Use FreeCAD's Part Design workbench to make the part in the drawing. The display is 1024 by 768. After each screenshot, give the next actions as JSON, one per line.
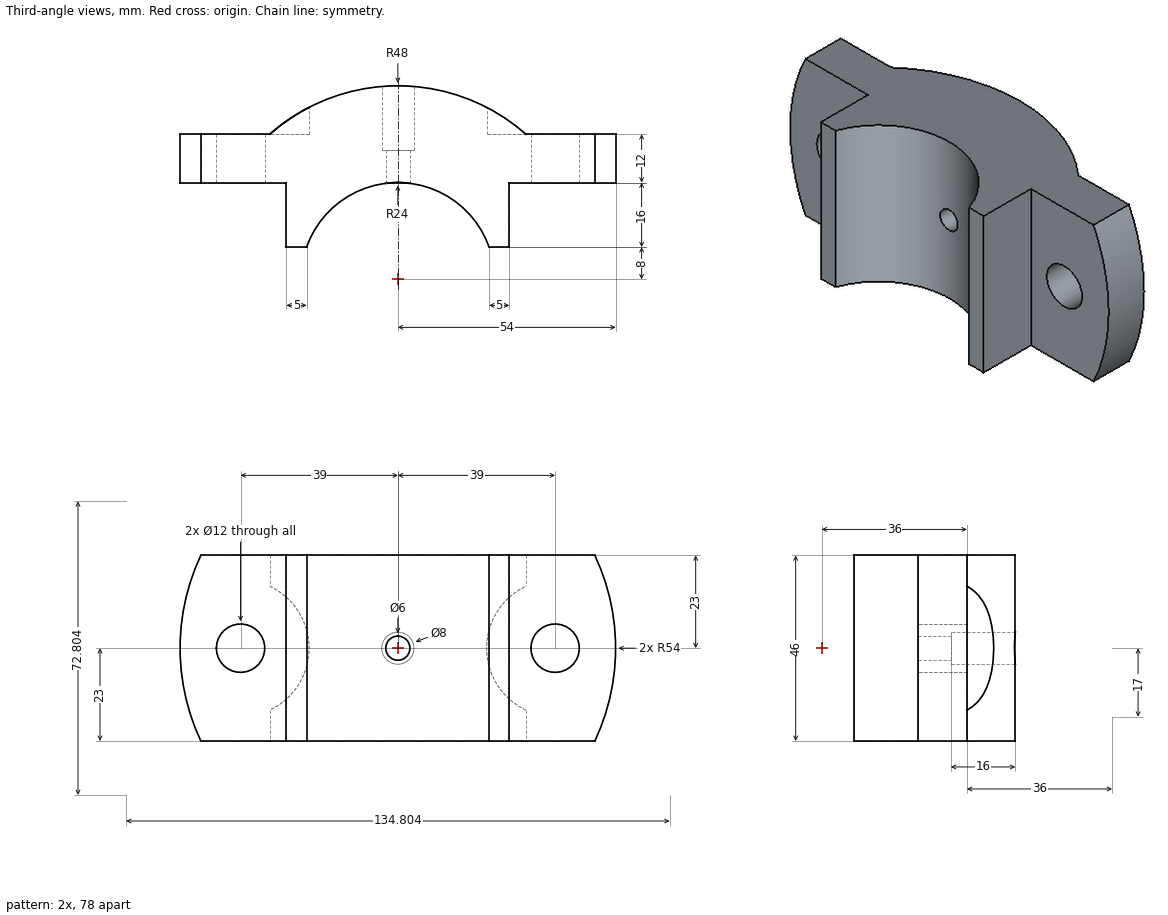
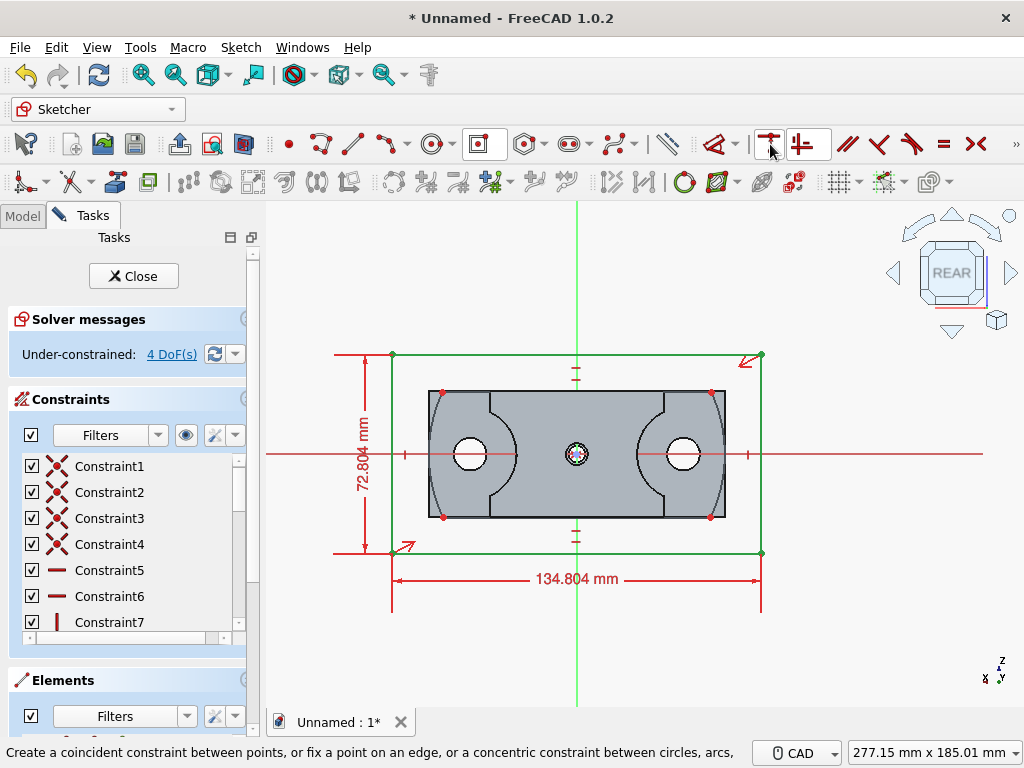
{"action": "left_click", "coordinate": [431, 429]}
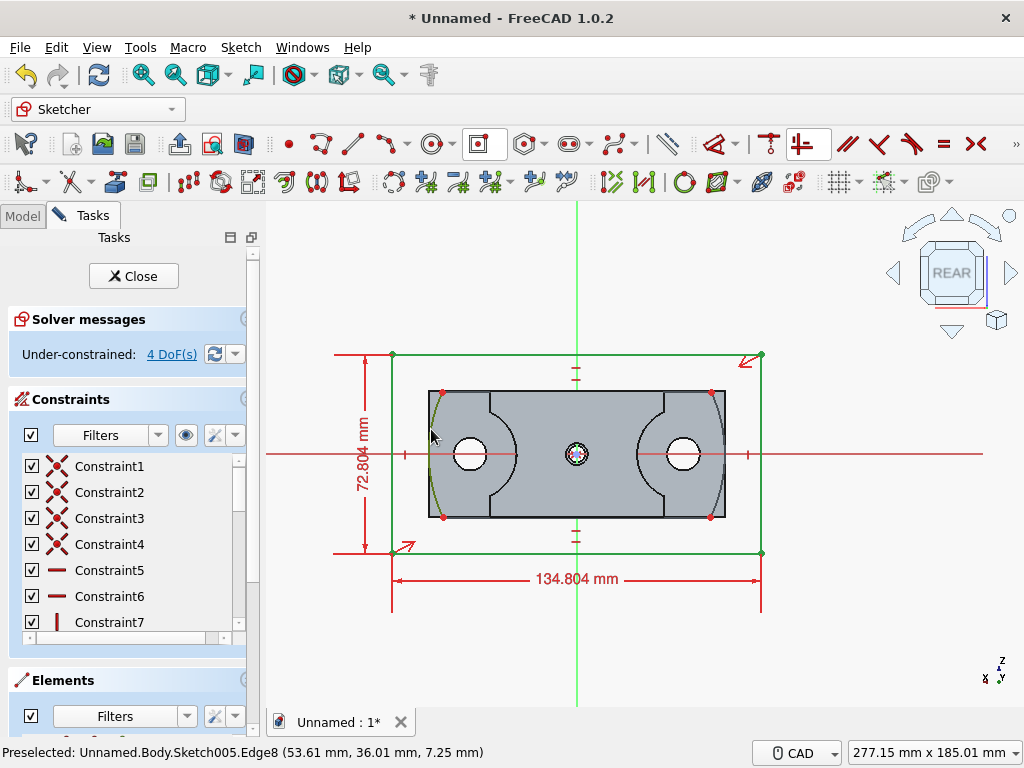
{"action": "left_click", "coordinate": [722, 481]}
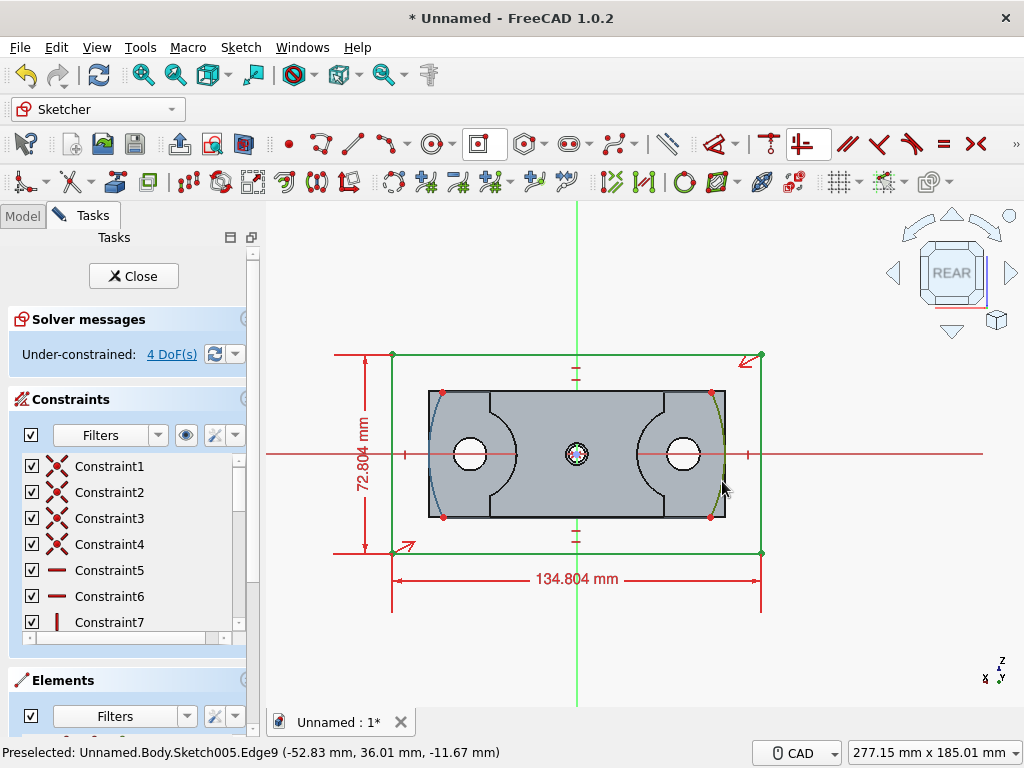
{"action": "left_click", "coordinate": [944, 144]}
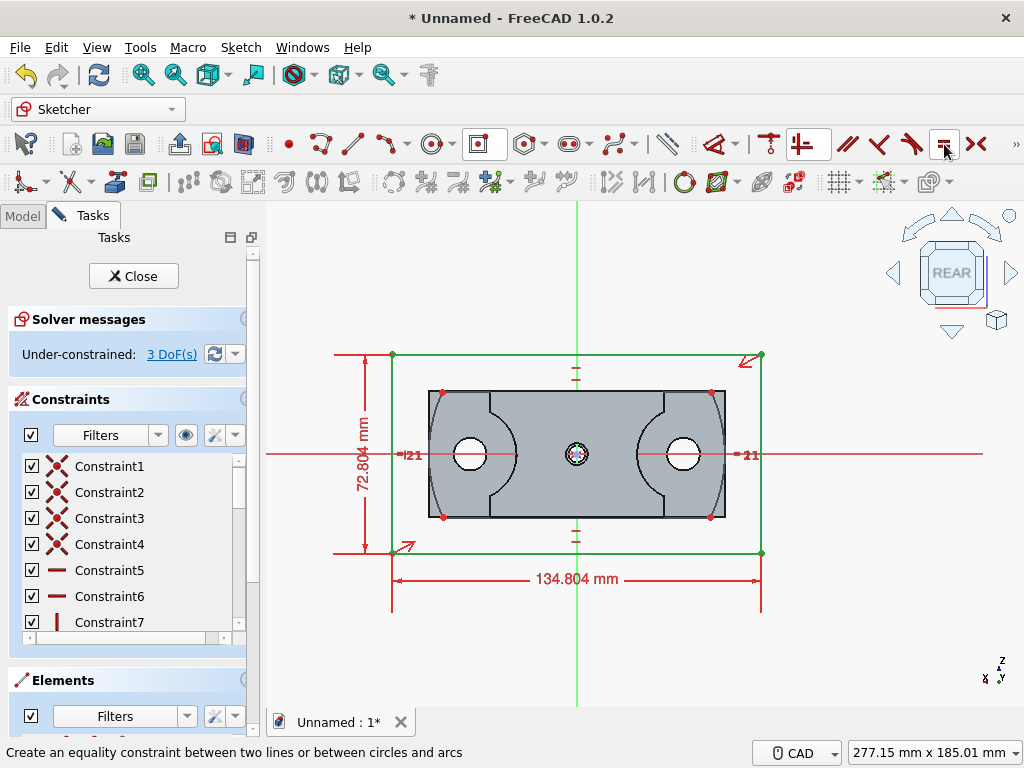
{"action": "left_click", "coordinate": [714, 144]}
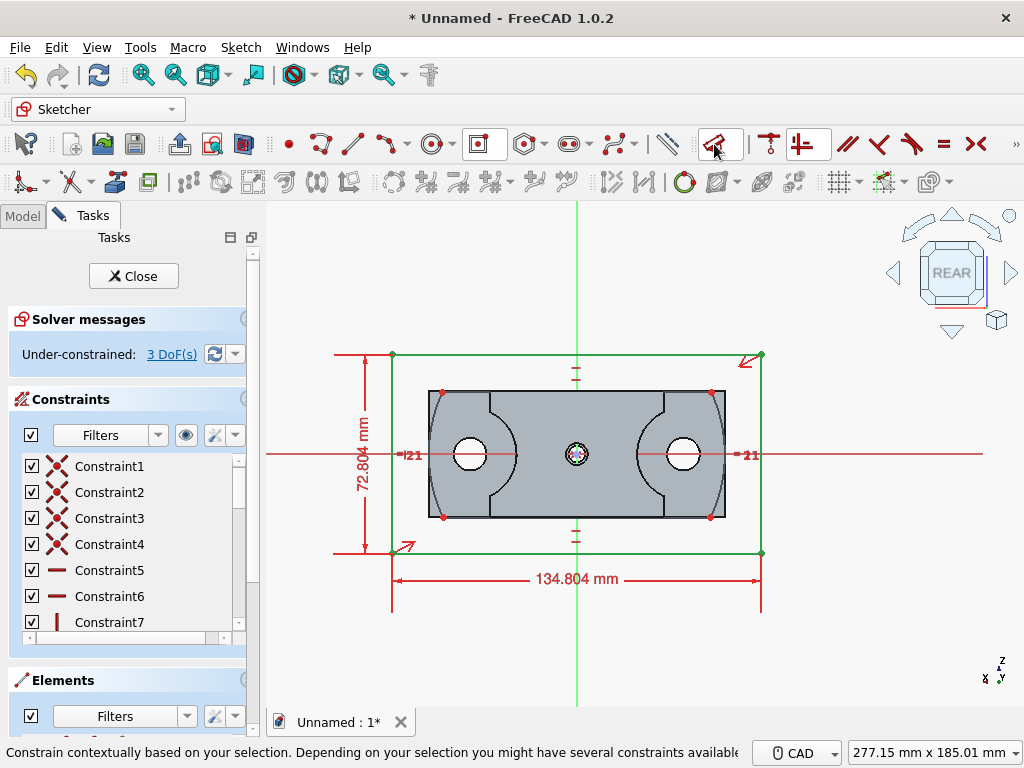
{"action": "left_click", "coordinate": [431, 429]}
{"action": "left_click", "coordinate": [407, 512]}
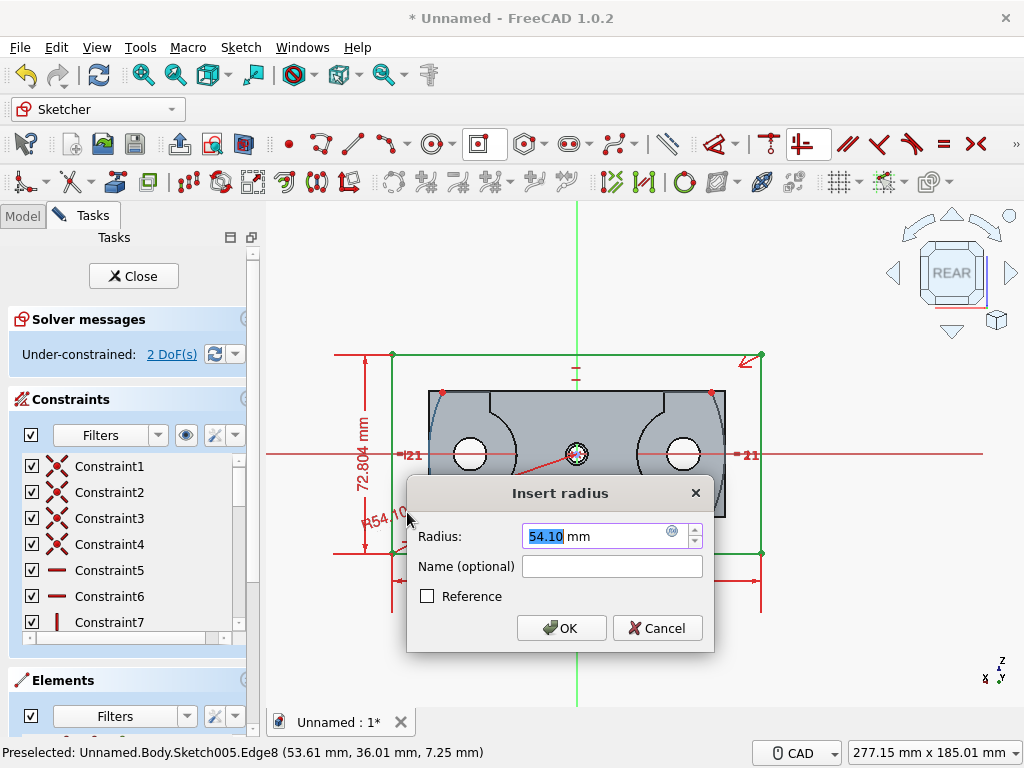
{"action": "type", "text": "54"}
{"action": "key", "text": "Return"}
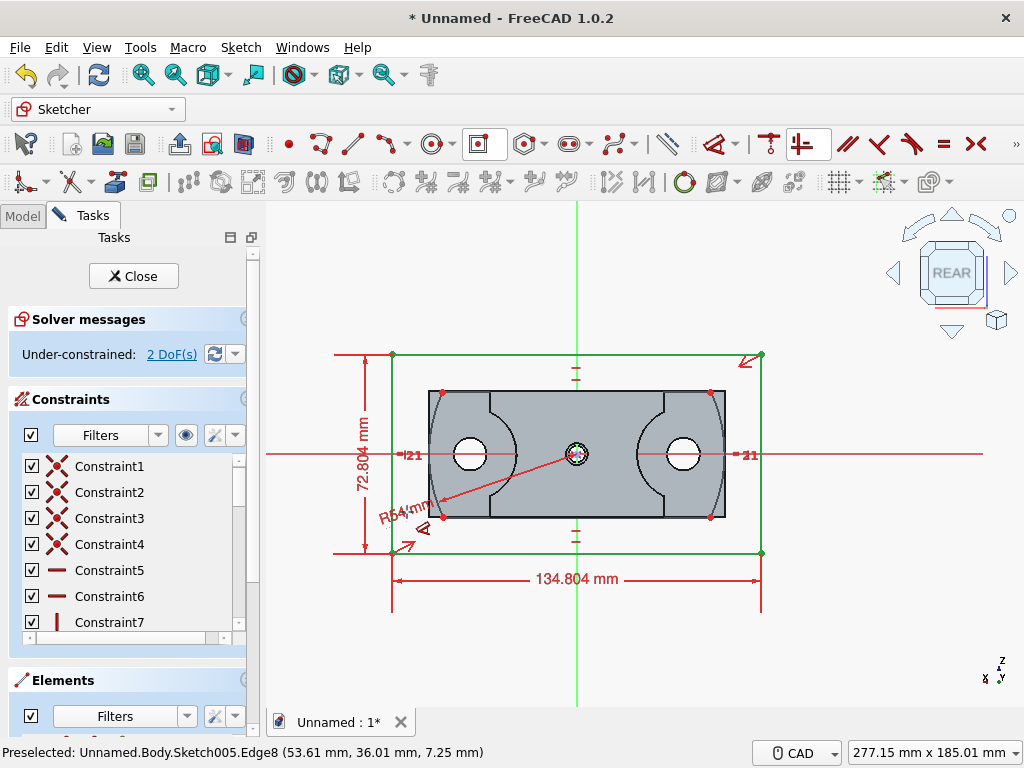
{"action": "left_click", "coordinate": [710, 518]}
{"action": "left_click", "coordinate": [744, 486]}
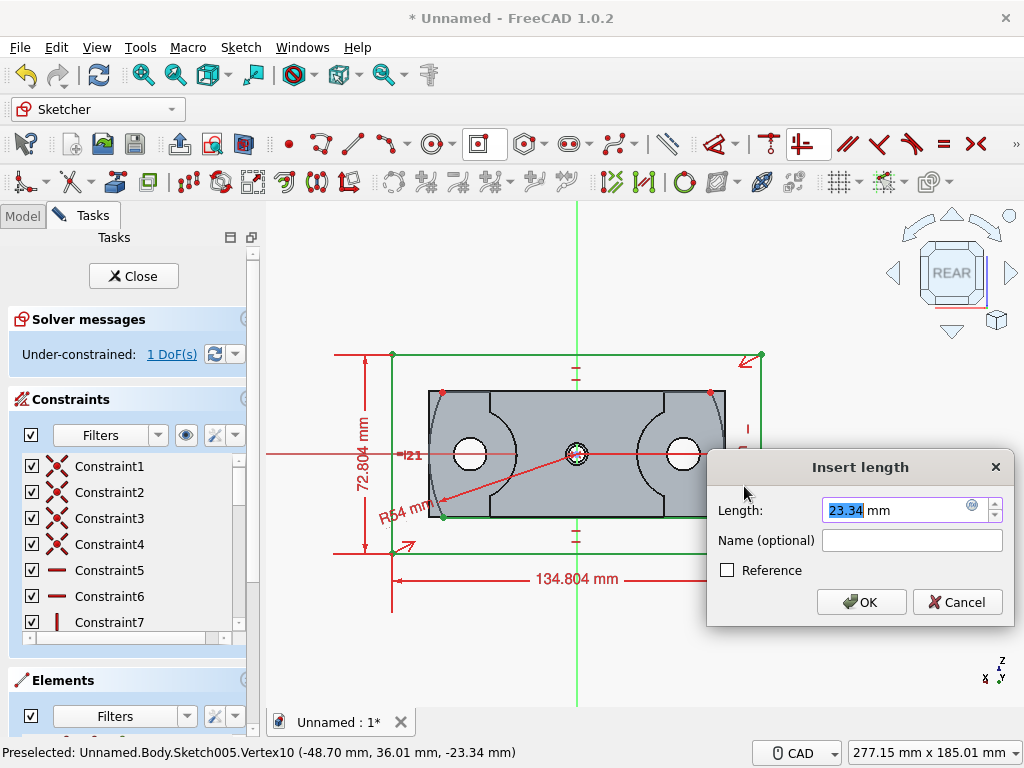
{"action": "type", "text": "23"}
{"action": "key", "text": "Return"}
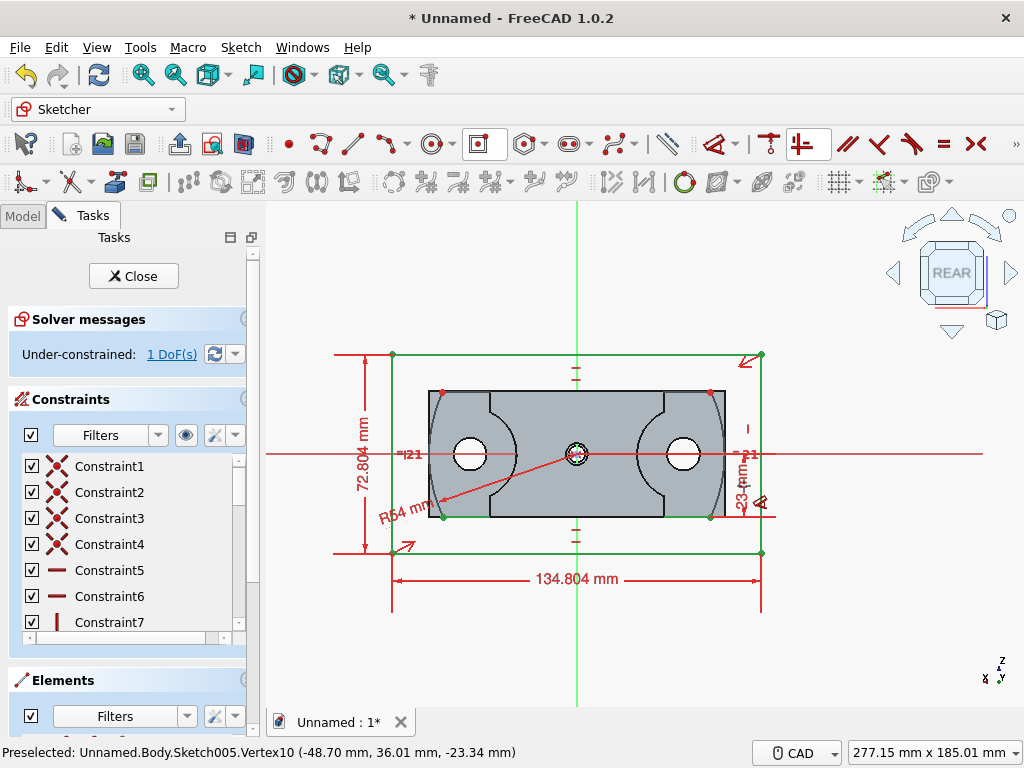
{"action": "left_click", "coordinate": [443, 392]}
{"action": "left_click", "coordinate": [409, 423]}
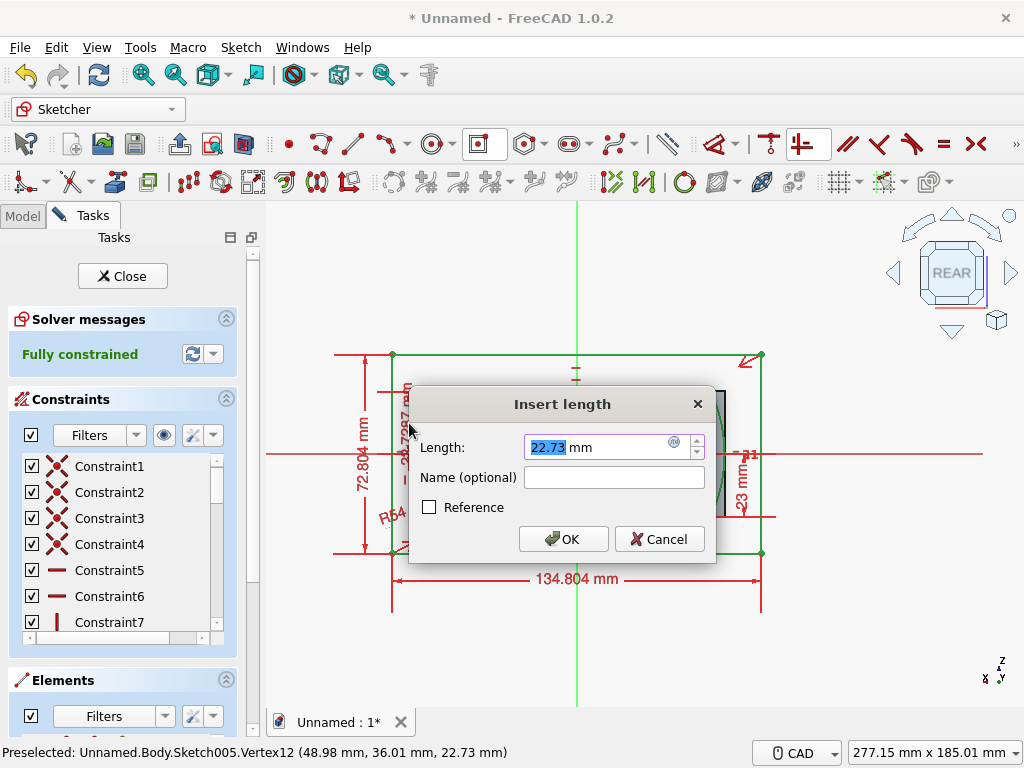
{"action": "type", "text": "23"}
{"action": "key", "text": "Return"}
{"action": "key", "text": "Escape"}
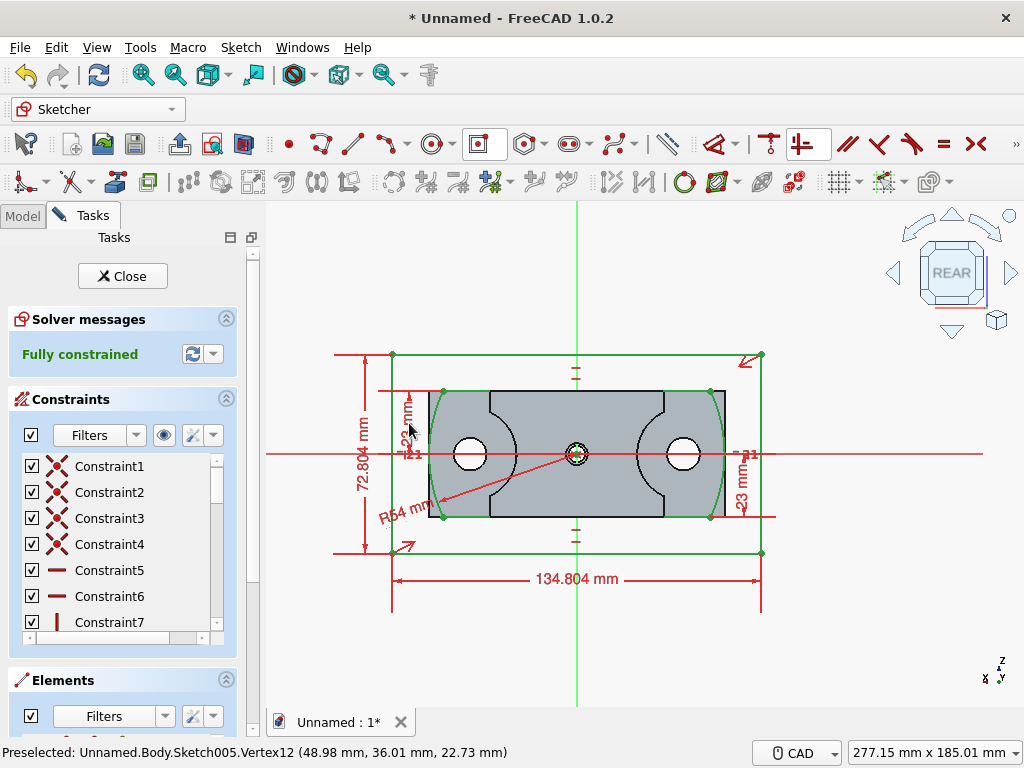
{"action": "left_click", "coordinate": [123, 276]}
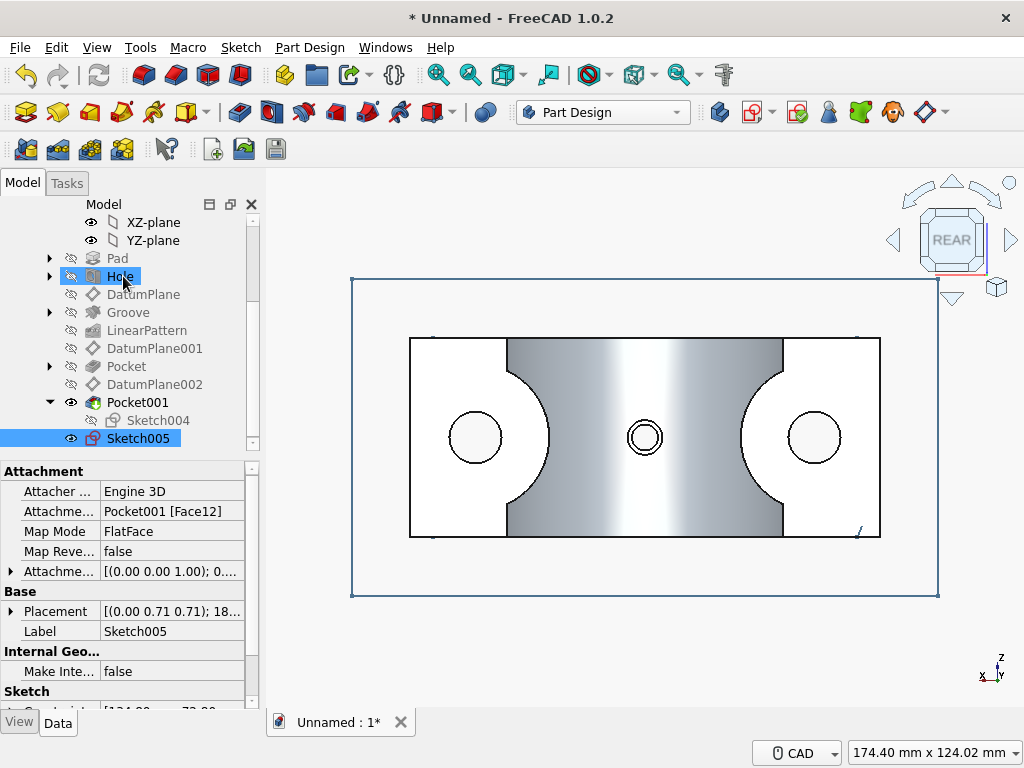
{"action": "left_click", "coordinate": [240, 112]}